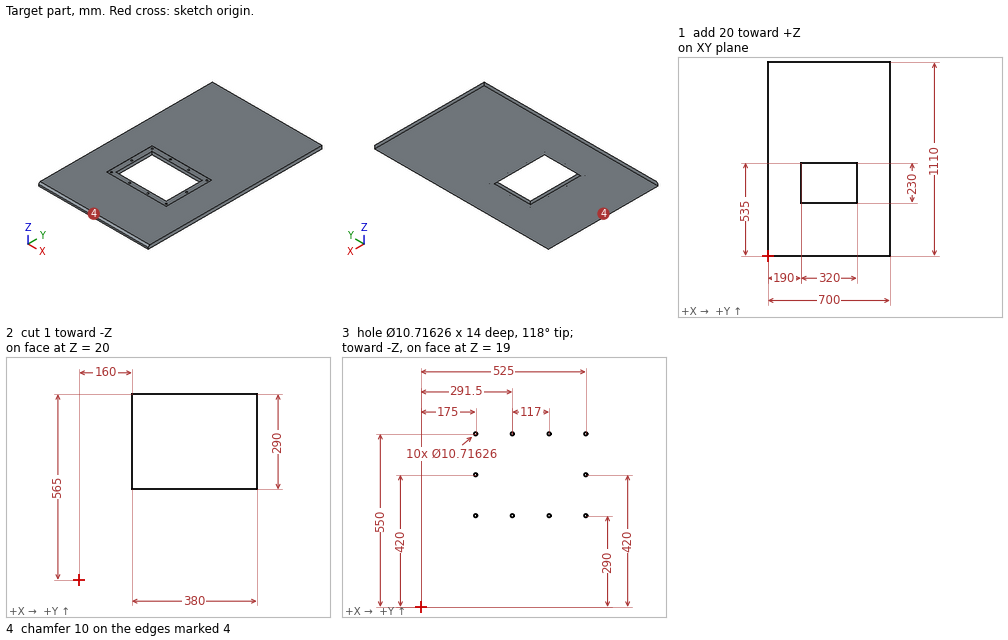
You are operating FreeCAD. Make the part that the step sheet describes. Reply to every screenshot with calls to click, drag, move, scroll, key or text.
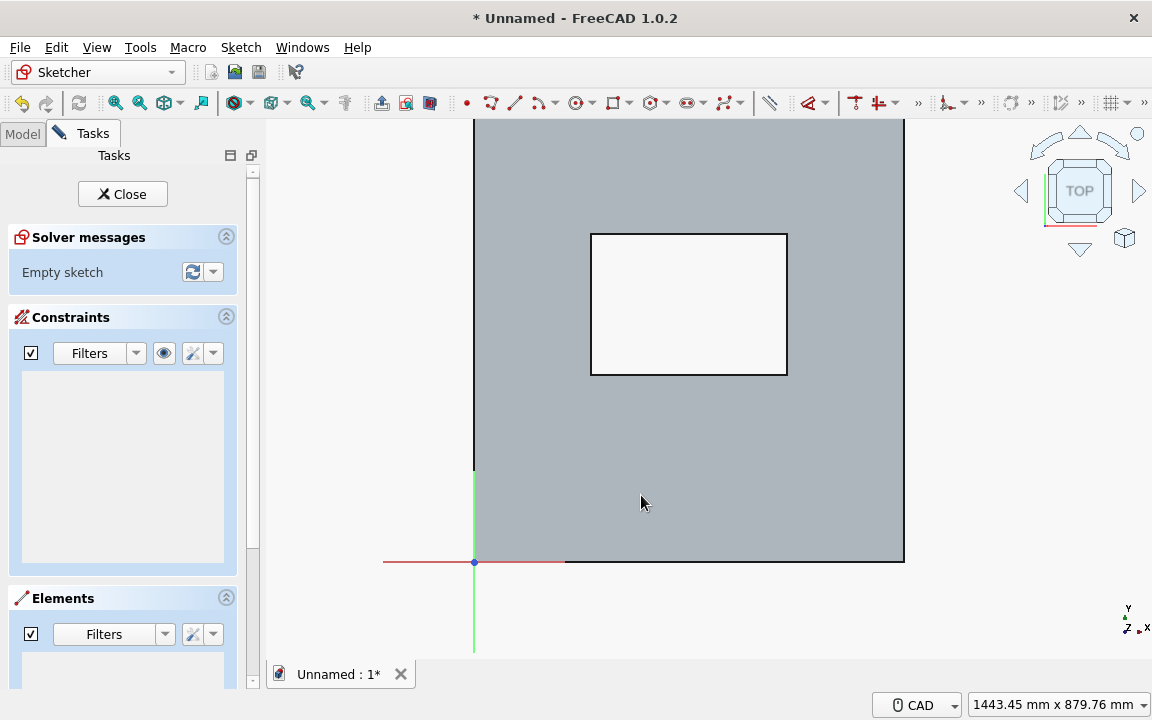
click(614, 104)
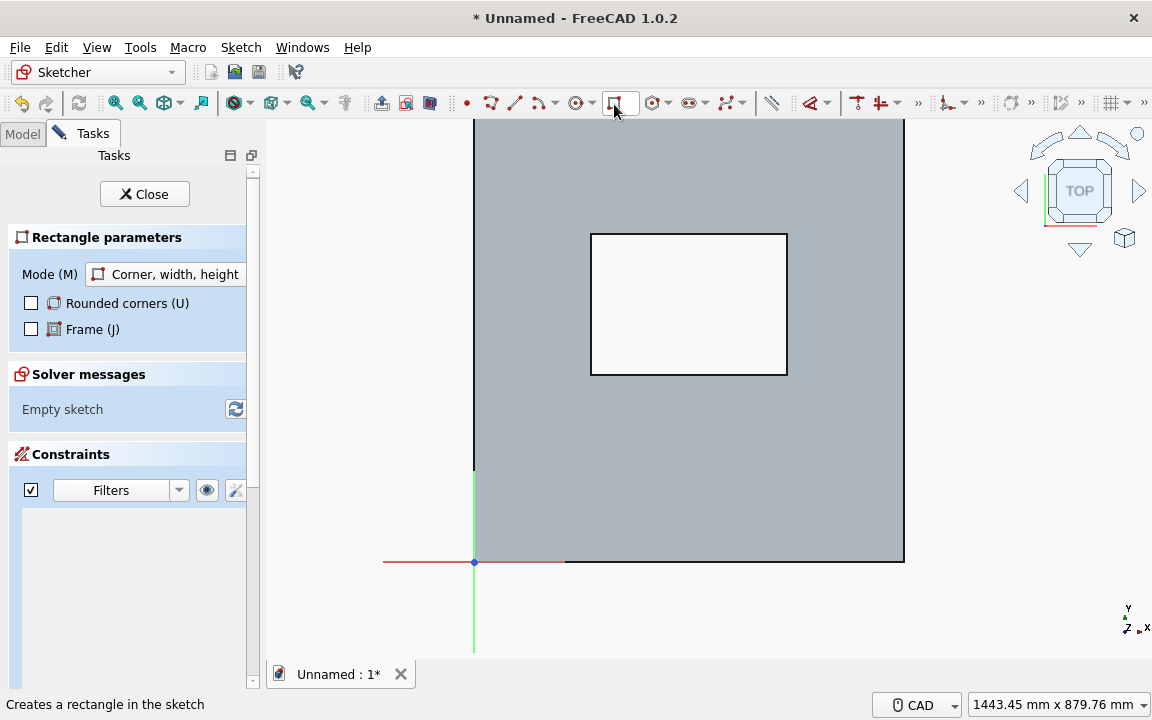
click(572, 215)
move(806, 393)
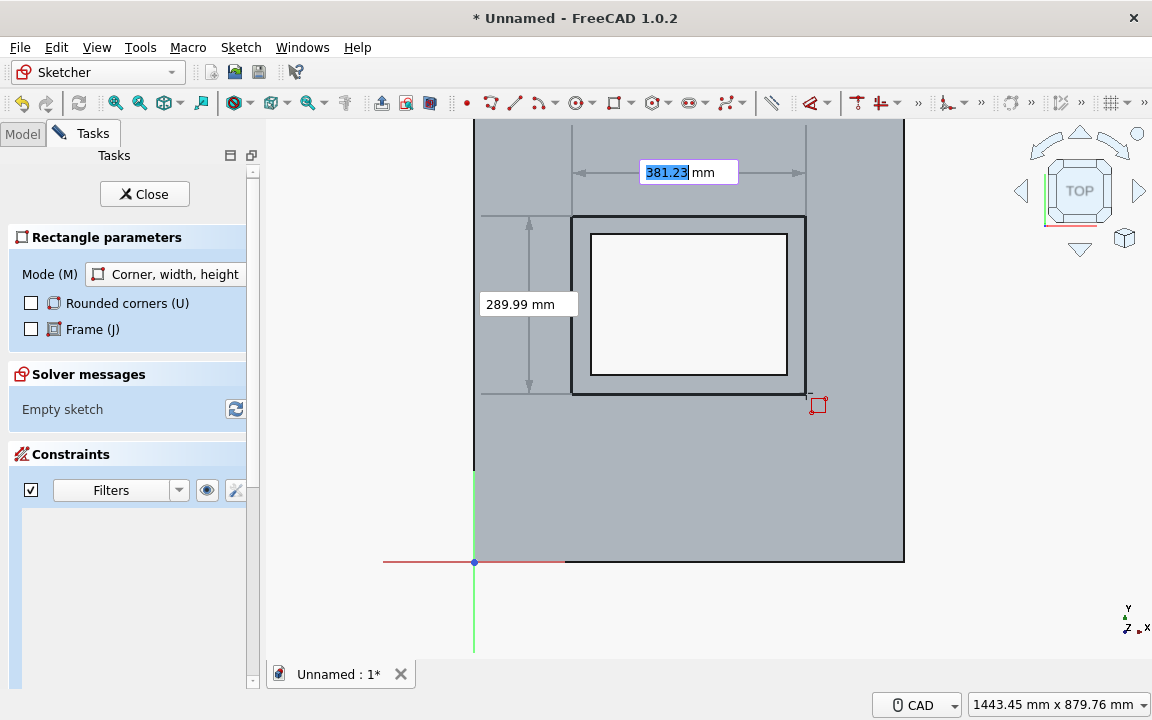
text(380)
key(Tab)
text(290)
key(Return)
key(Escape)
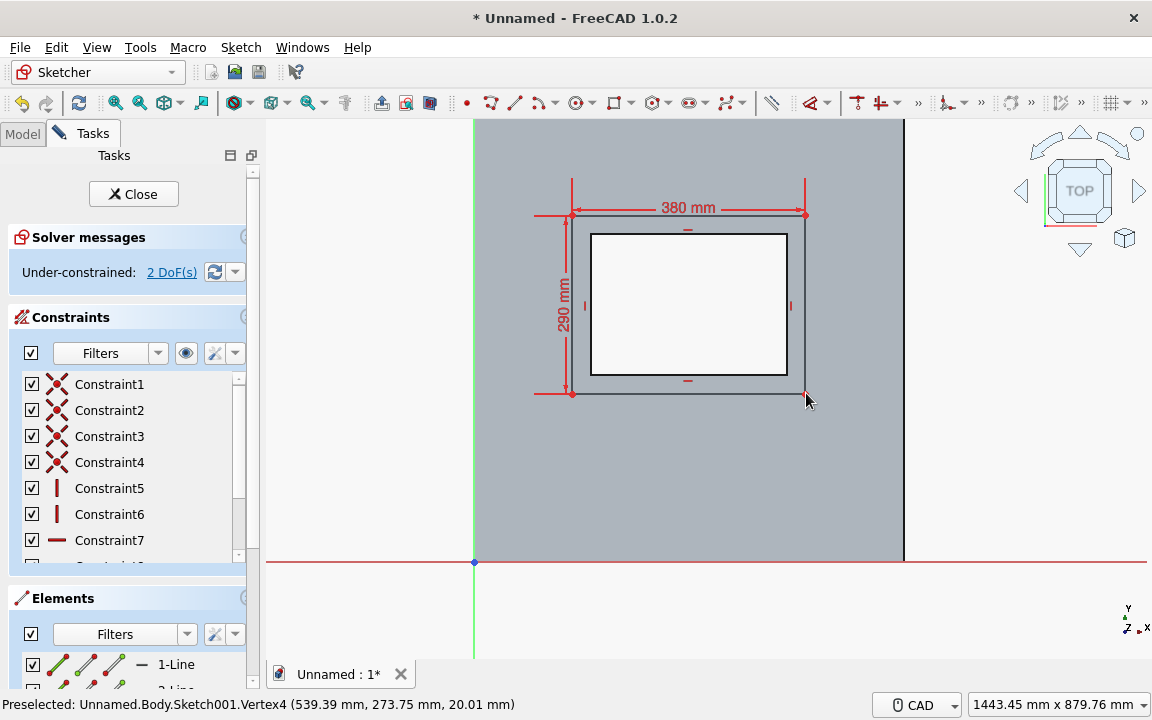
click(810, 104)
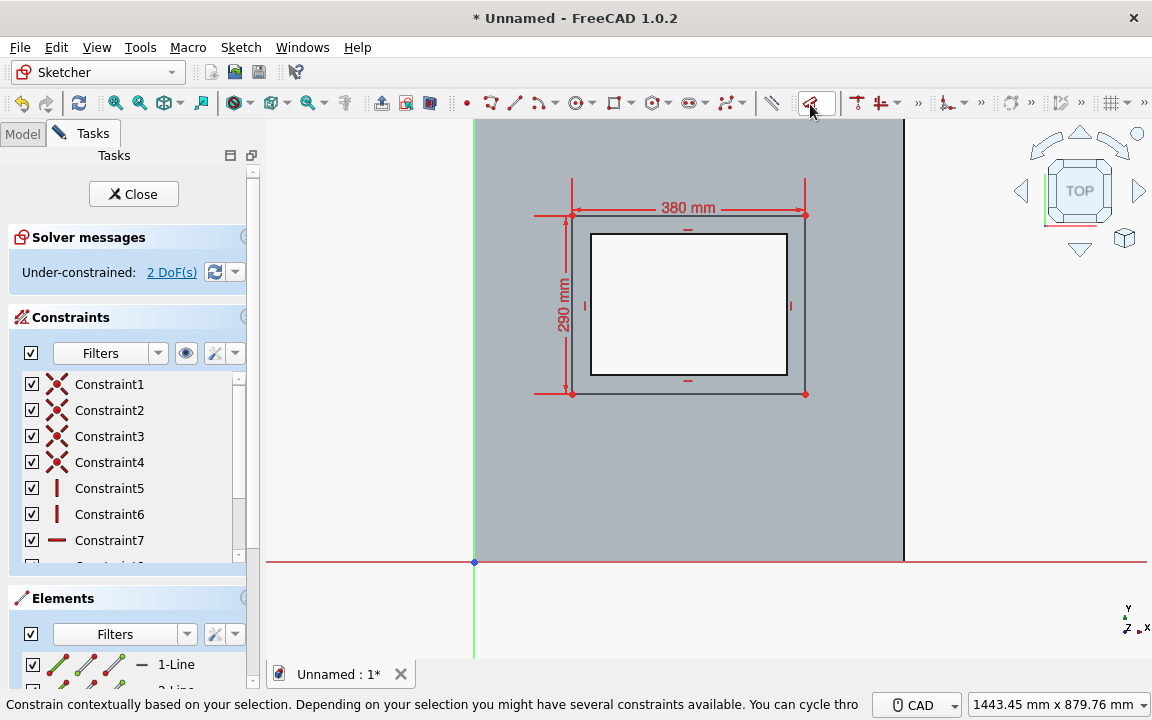
click(572, 216)
click(523, 596)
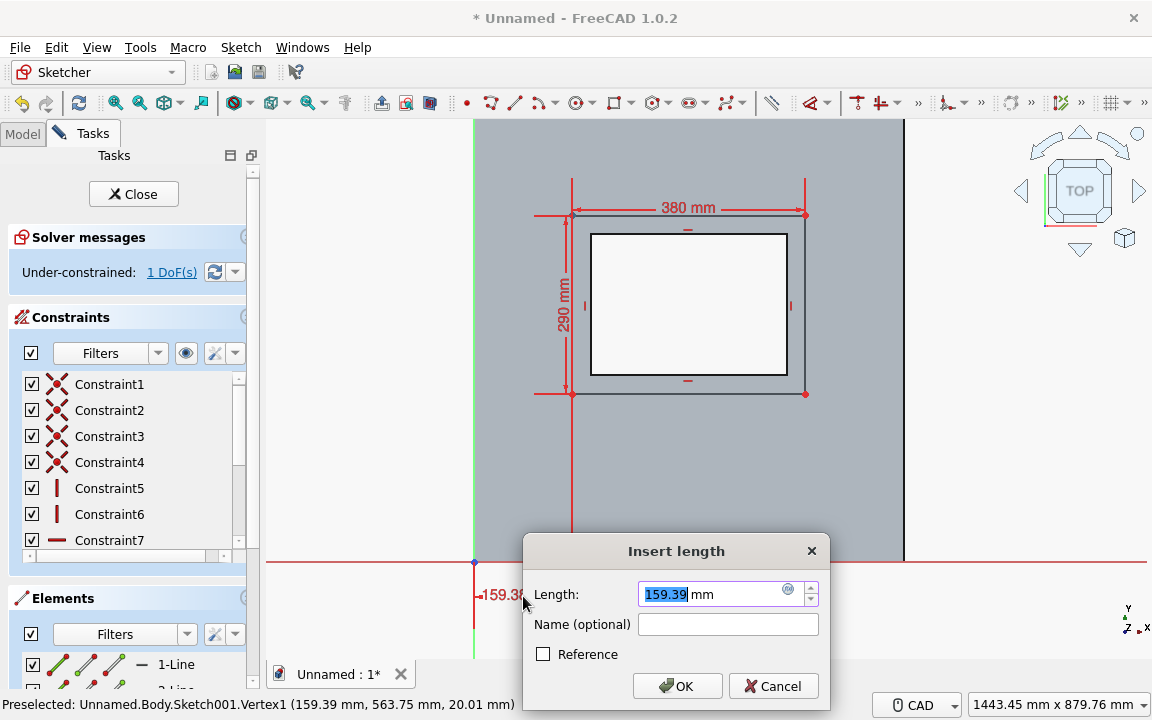
text(160)
key(Return)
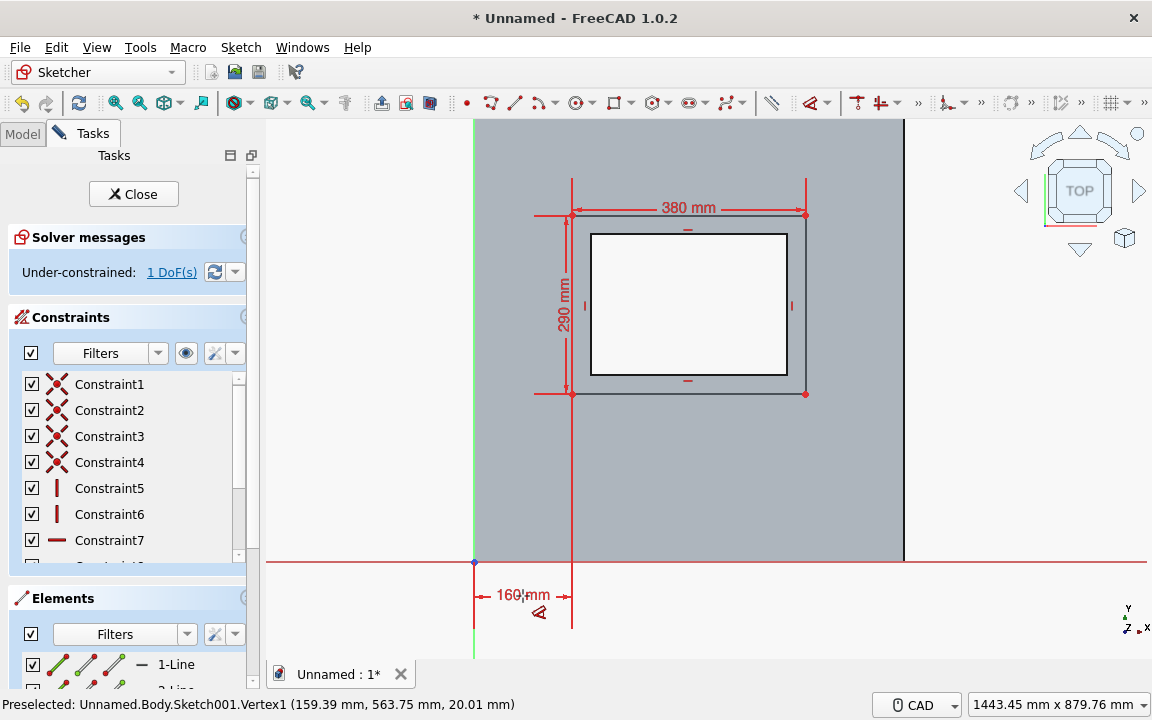
click(572, 216)
click(440, 389)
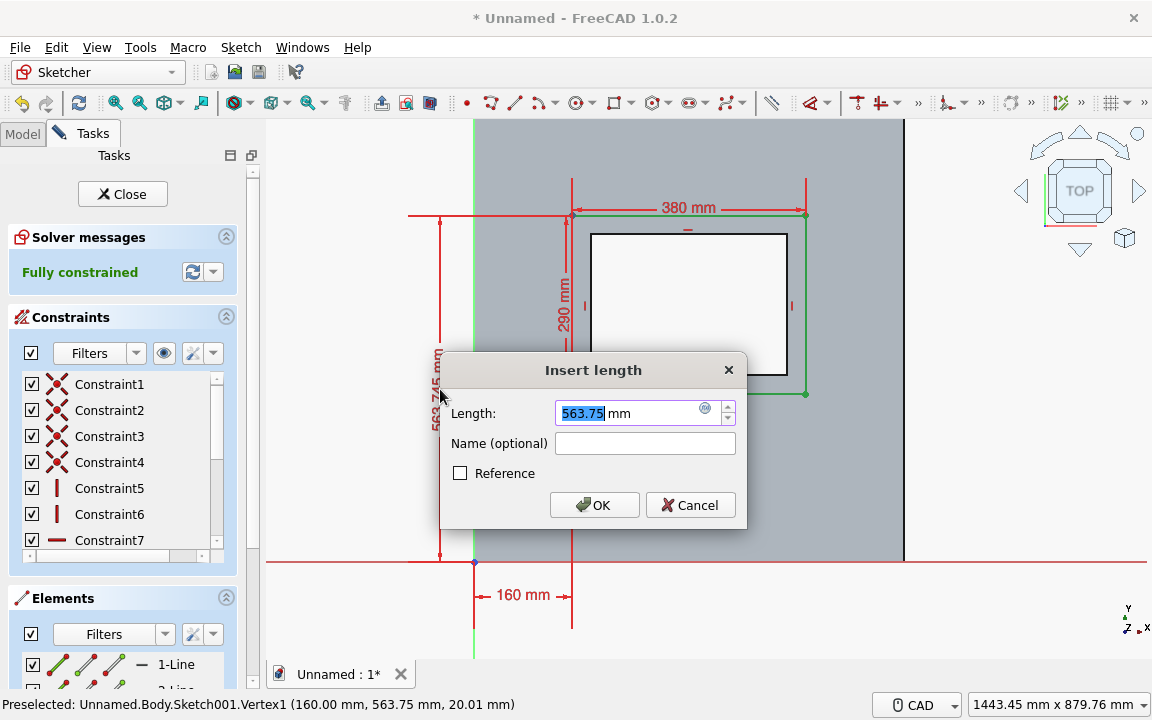
text(565)
key(Return)
key(Escape)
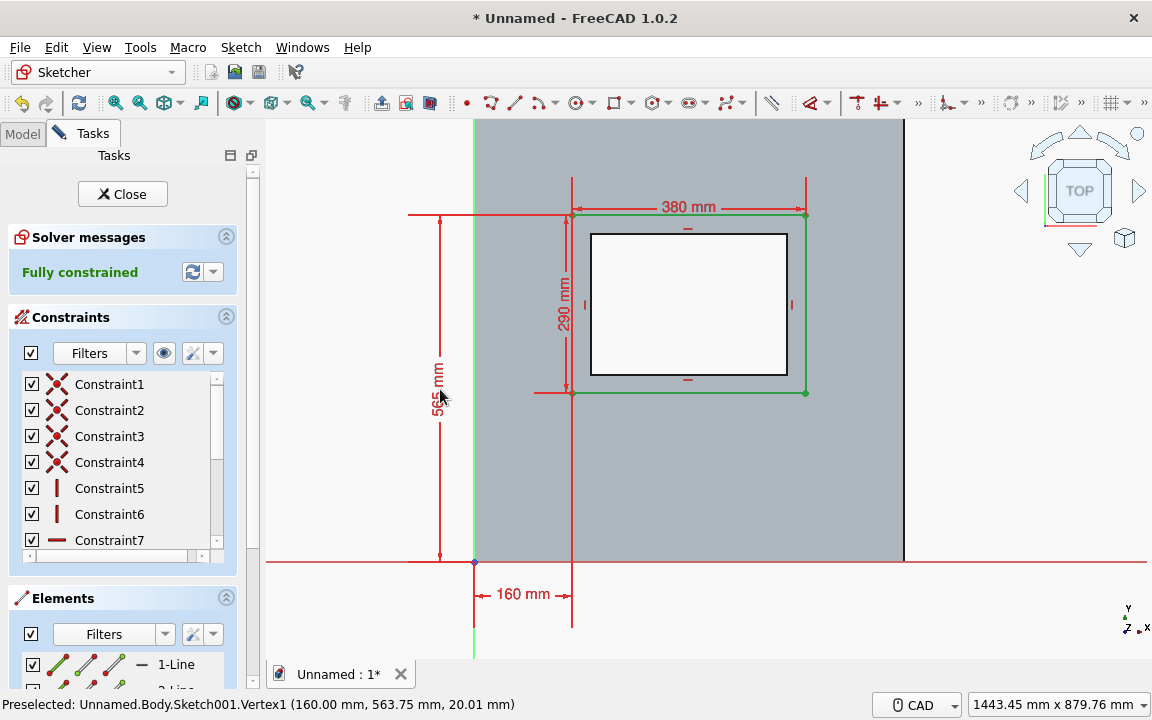
click(123, 194)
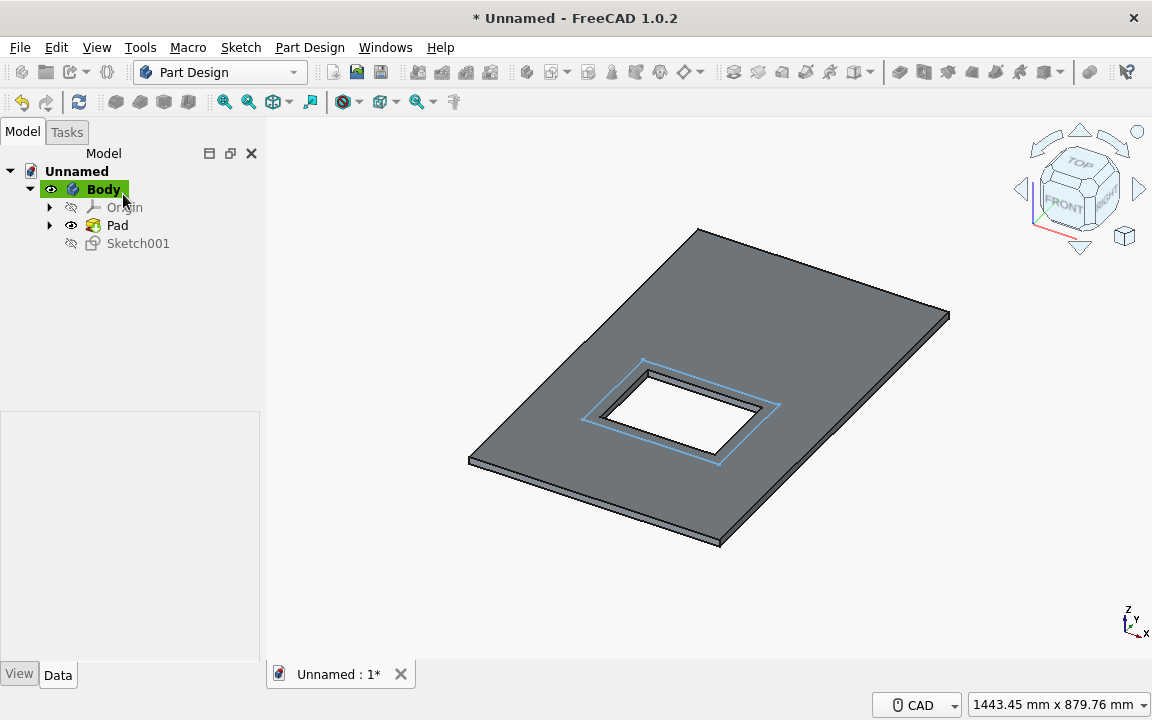
click(900, 72)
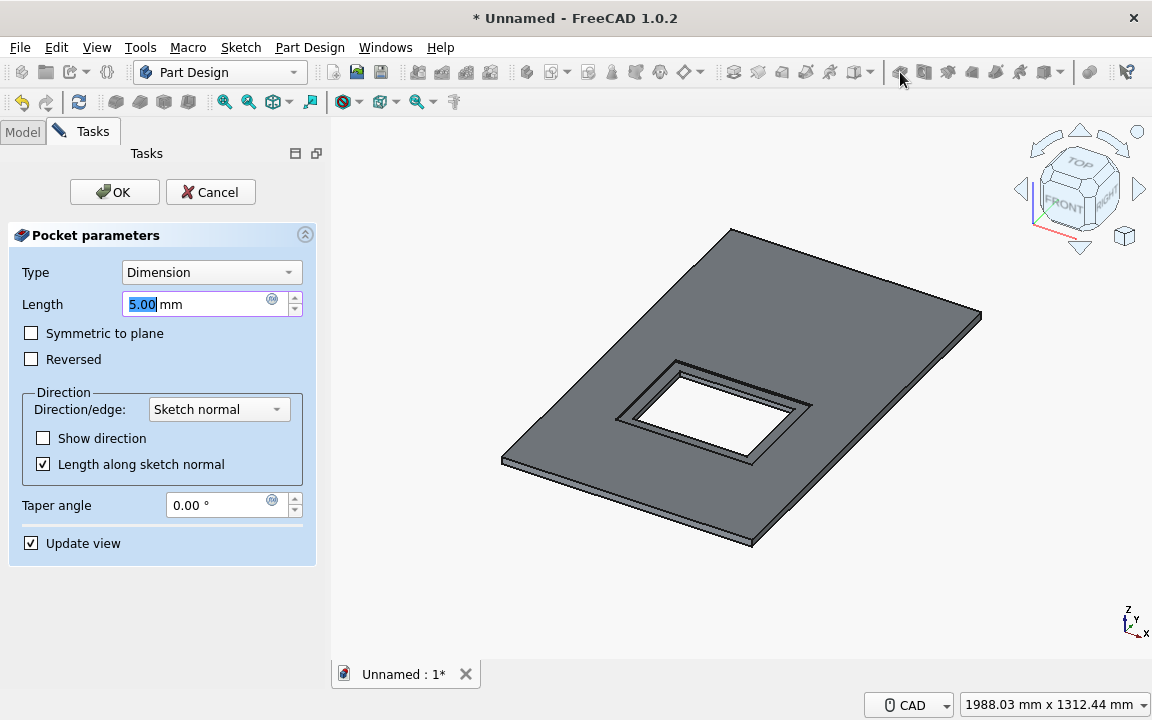
text(1)
key(Tab)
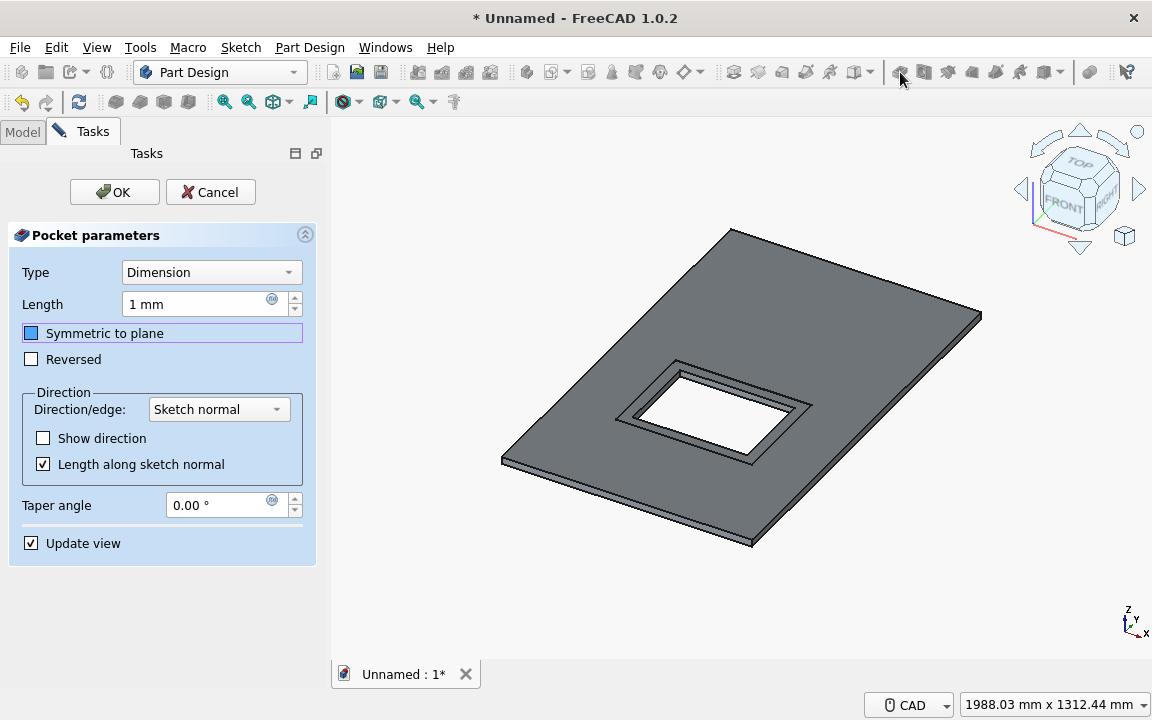
click(115, 192)